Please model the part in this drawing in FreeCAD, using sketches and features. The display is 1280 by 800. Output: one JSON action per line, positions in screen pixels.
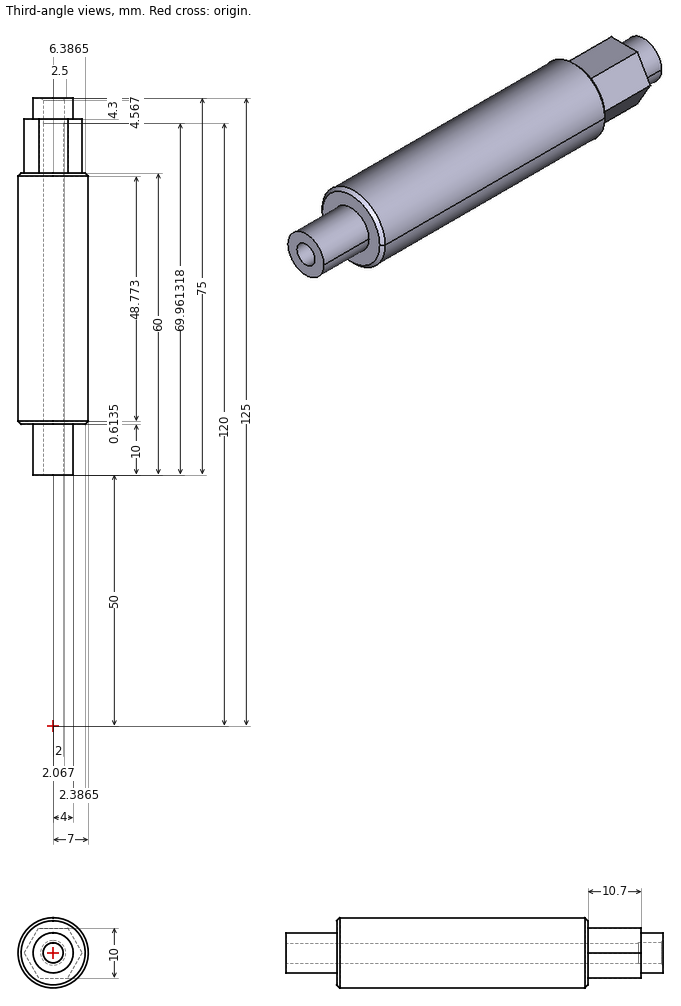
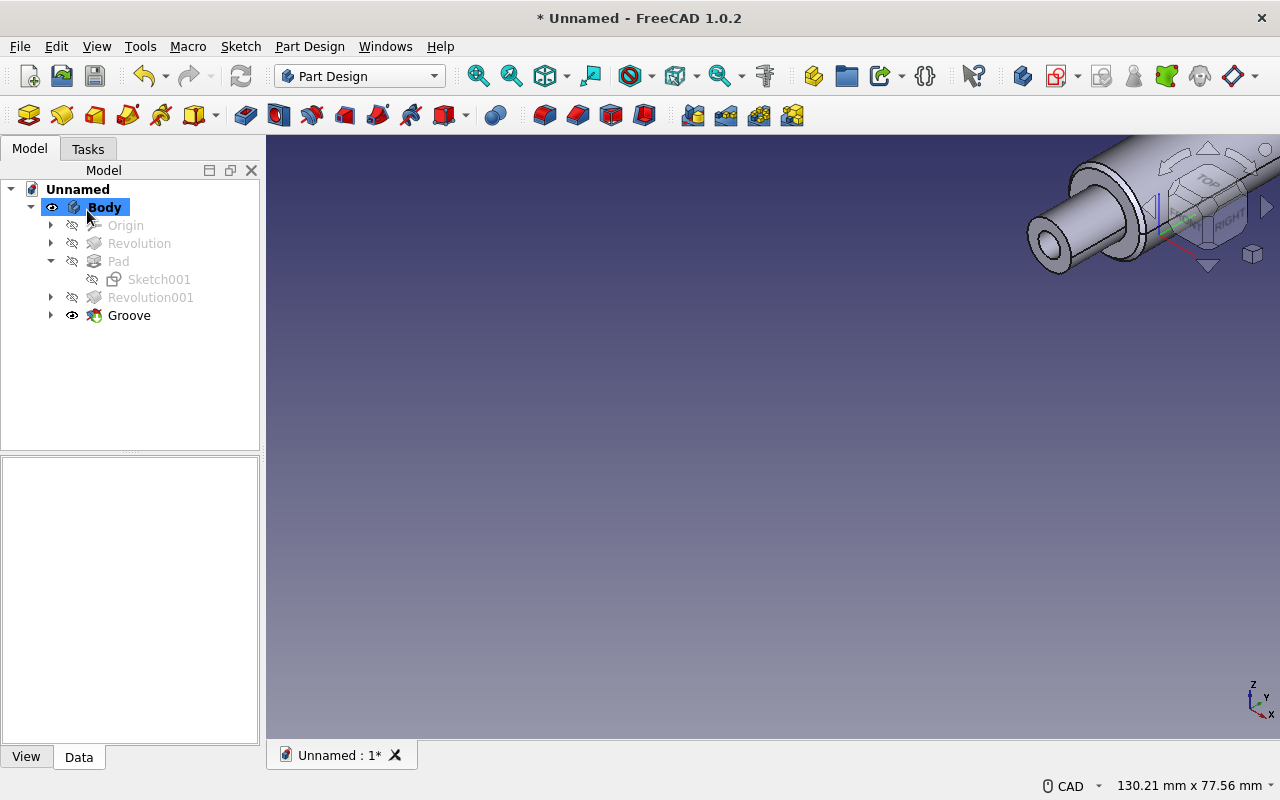
{"action": "key", "text": "v f"}